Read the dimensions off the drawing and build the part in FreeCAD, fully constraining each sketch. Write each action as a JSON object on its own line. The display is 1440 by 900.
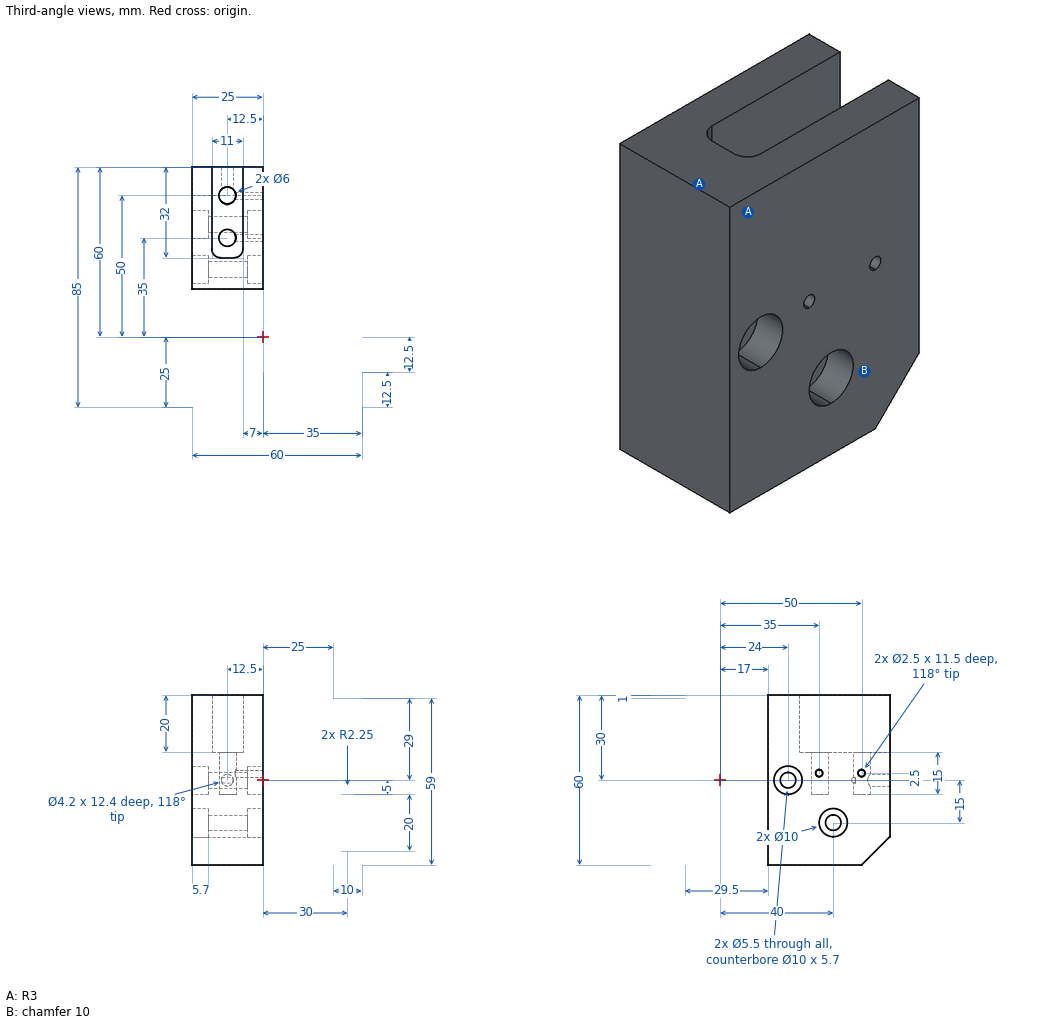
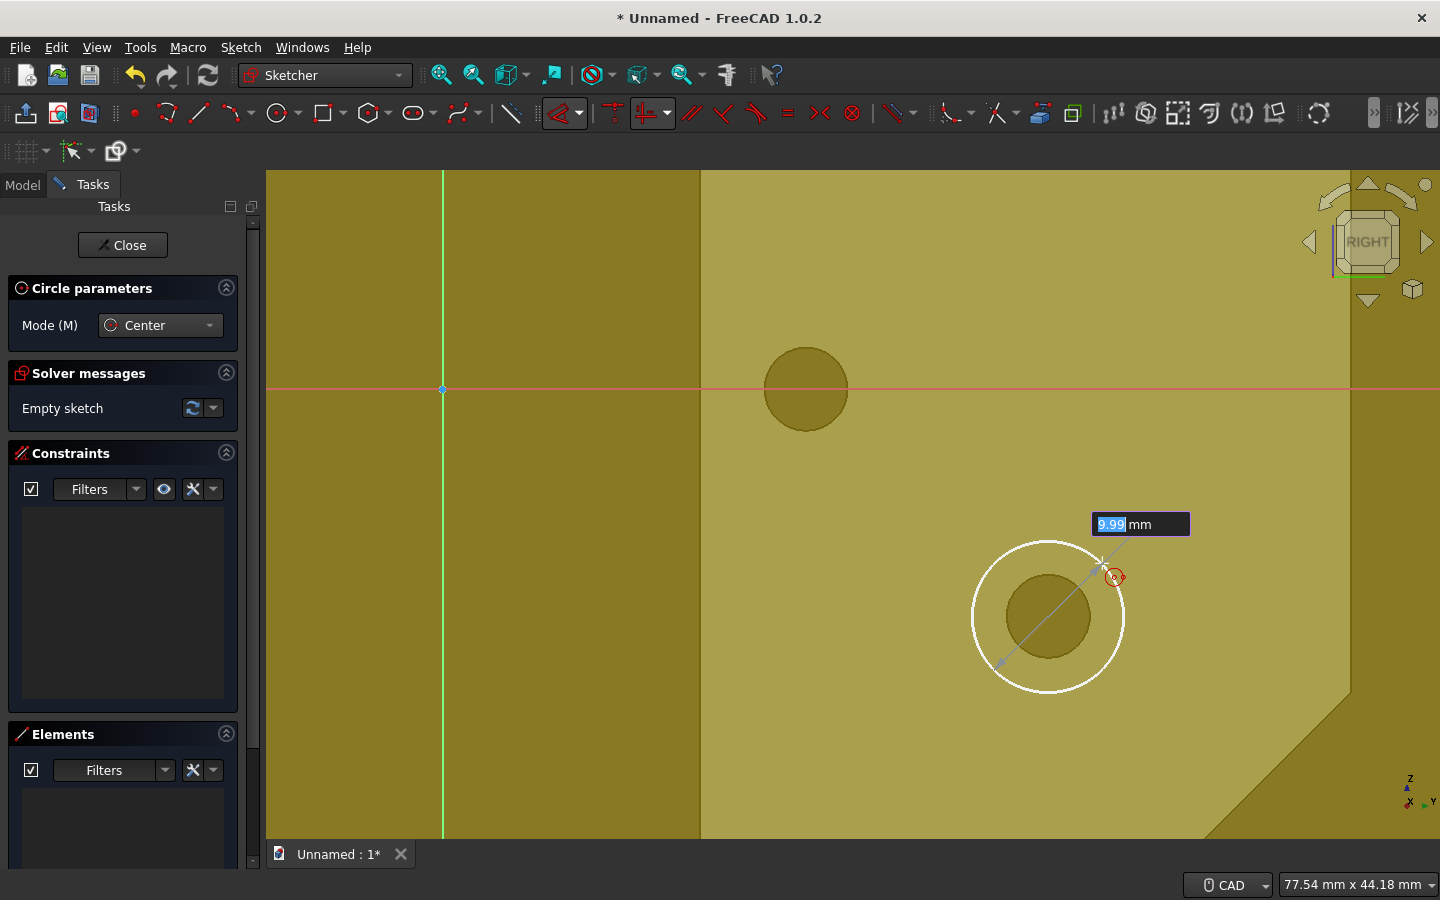
{"action": "type", "text": "10"}
{"action": "key", "text": "Return"}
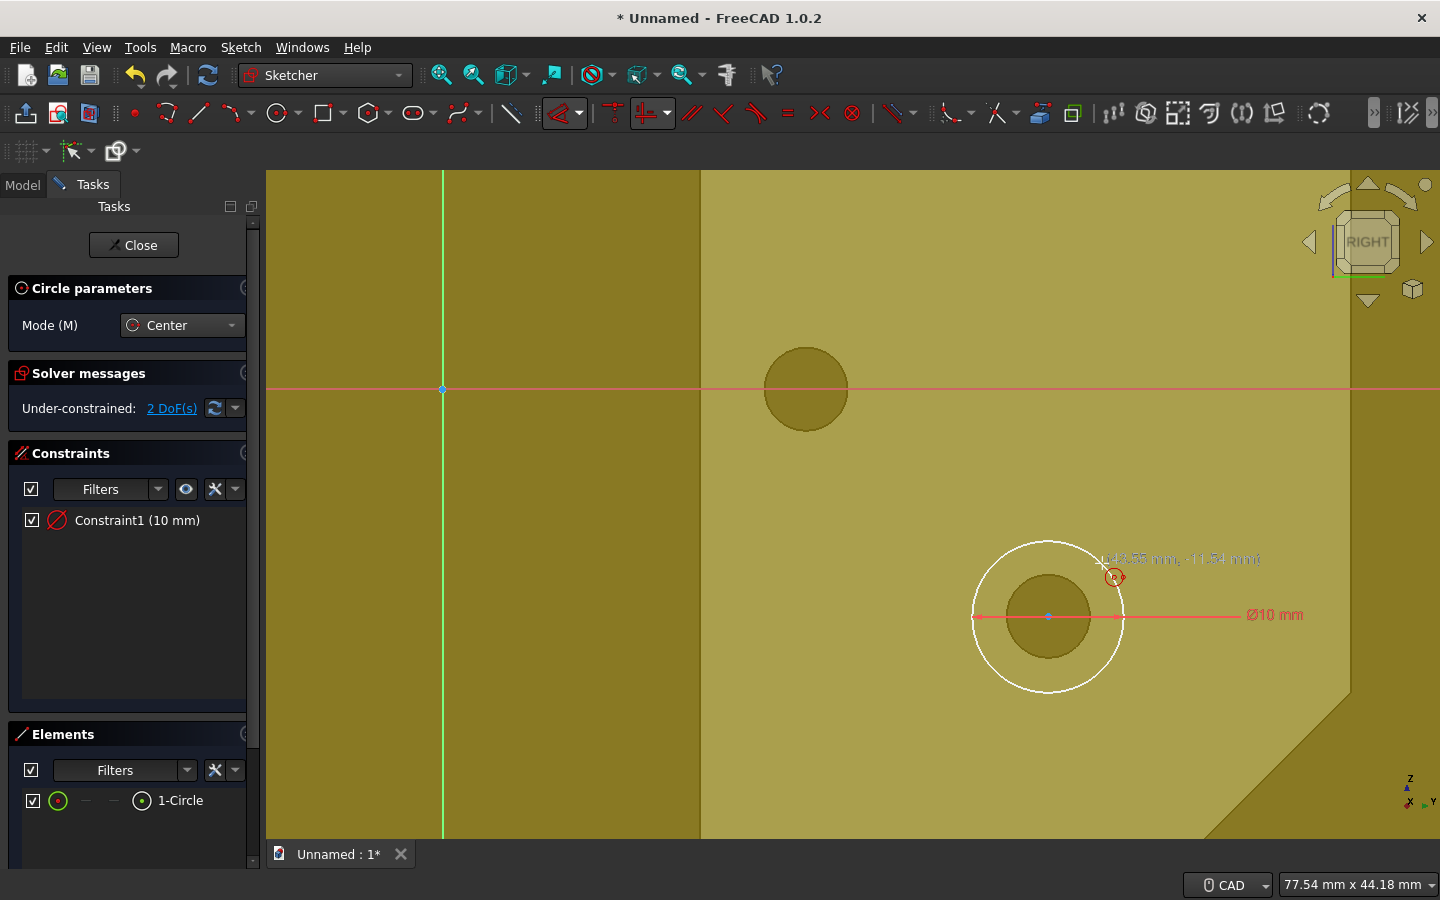
{"action": "left_click", "coordinate": [806, 389]}
{"action": "mouse_move", "coordinate": [860, 336]}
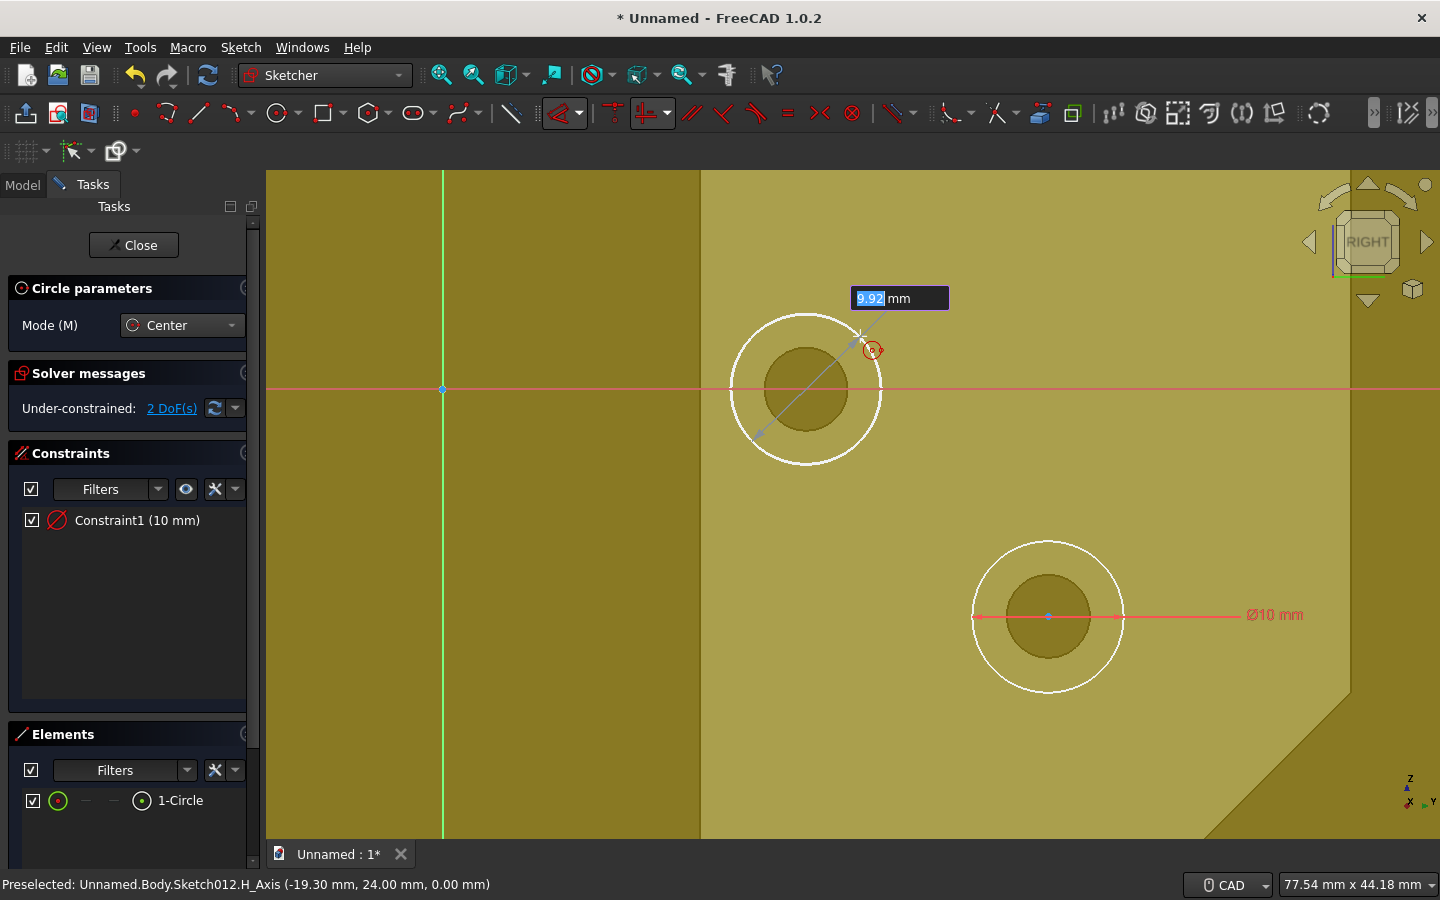
{"action": "type", "text": "10"}
{"action": "key", "text": "Return"}
{"action": "key", "text": "Escape"}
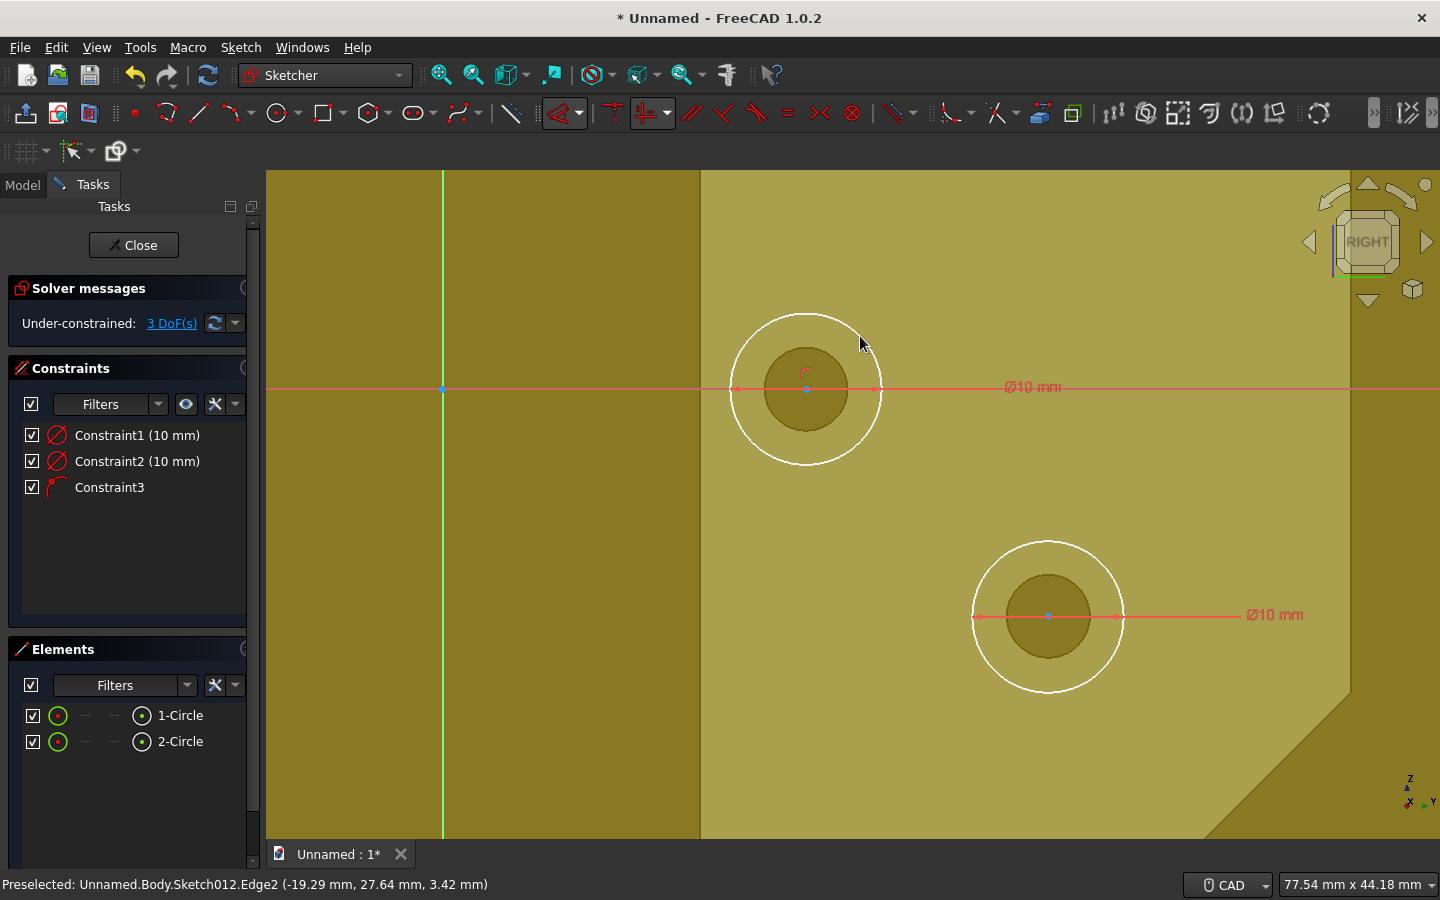
{"action": "left_click", "coordinate": [1048, 617]}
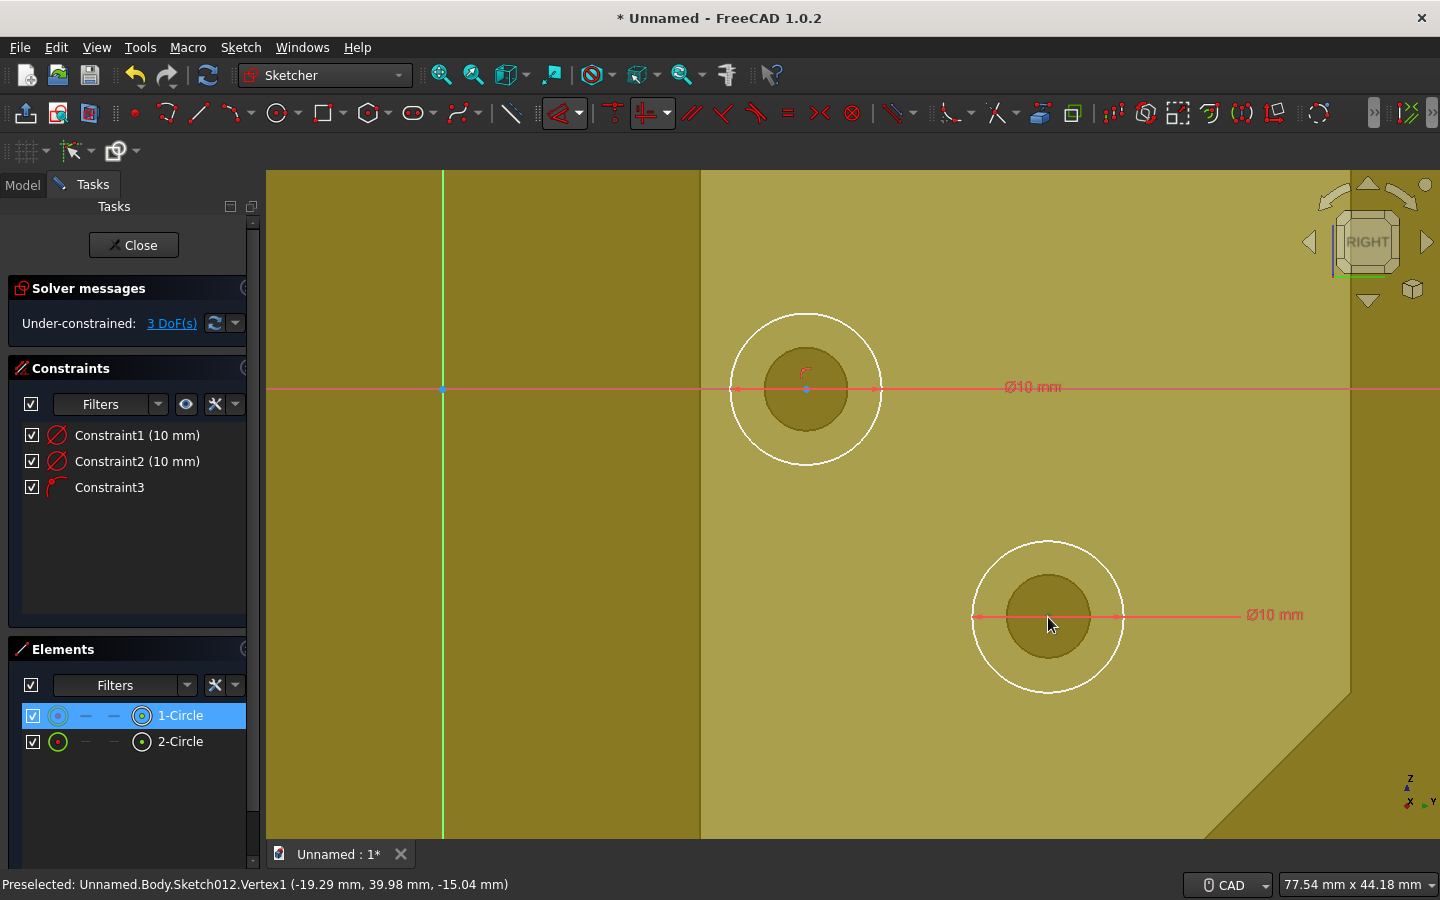
{"action": "left_click", "coordinate": [582, 114]}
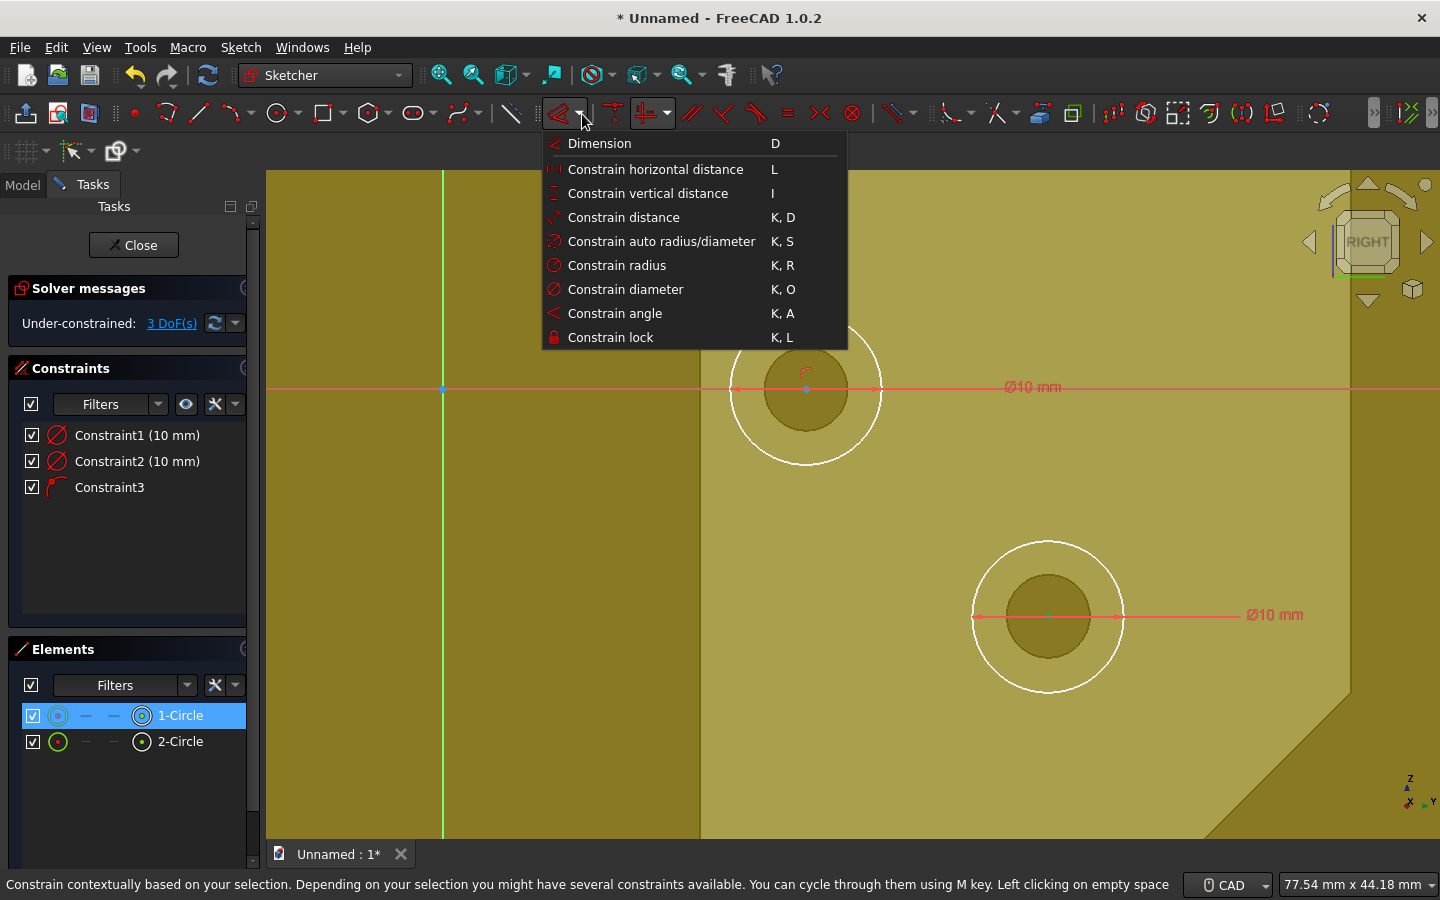
{"action": "left_click", "coordinate": [695, 169]}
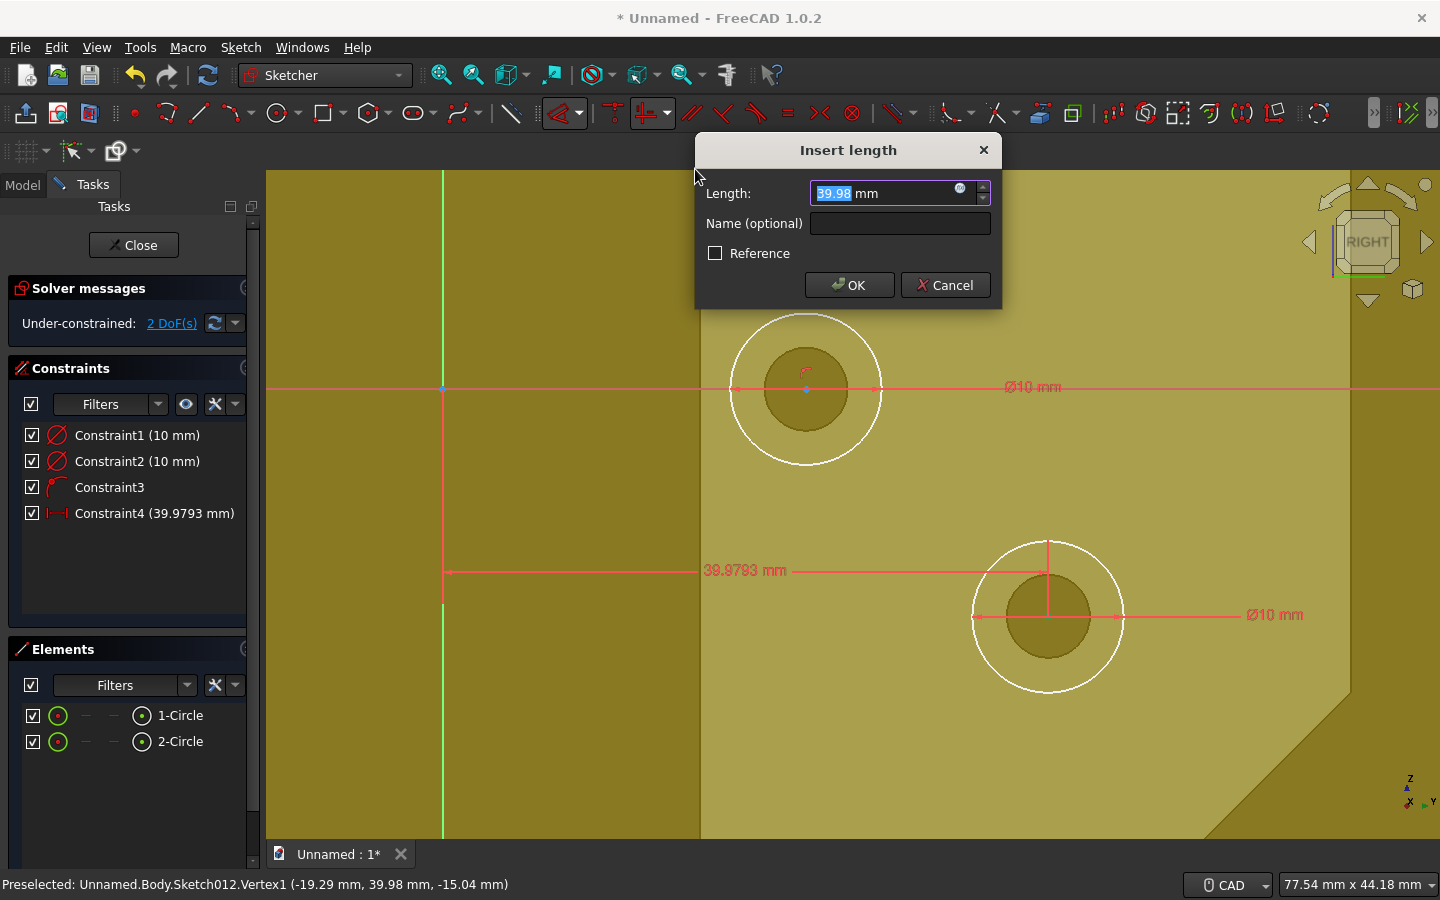
{"action": "type", "text": "40"}
{"action": "key", "text": "Return"}